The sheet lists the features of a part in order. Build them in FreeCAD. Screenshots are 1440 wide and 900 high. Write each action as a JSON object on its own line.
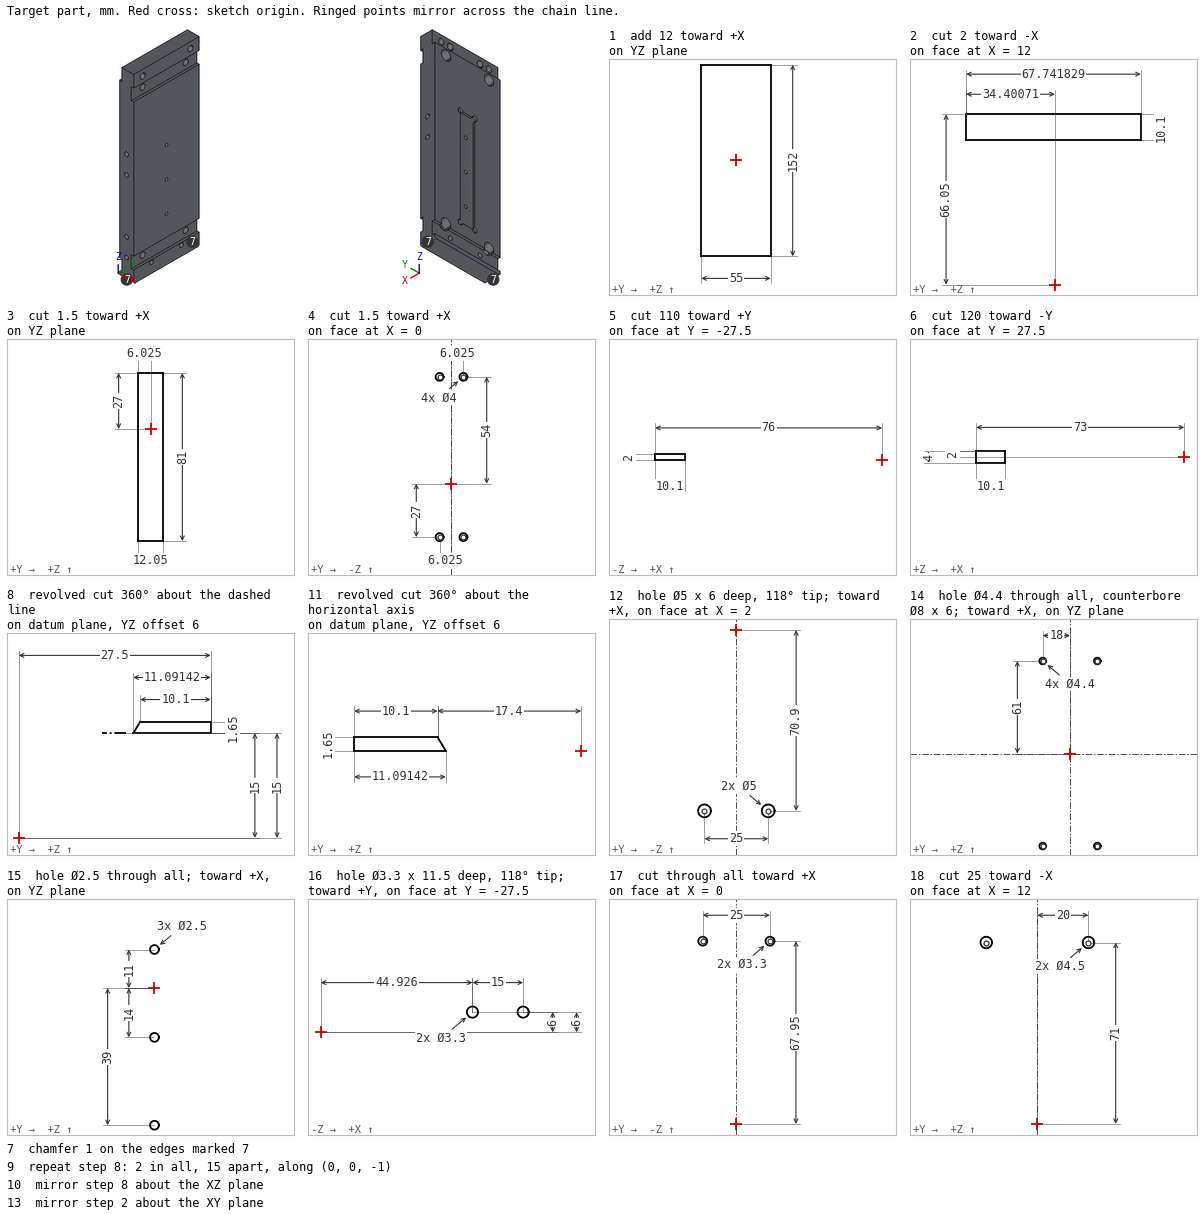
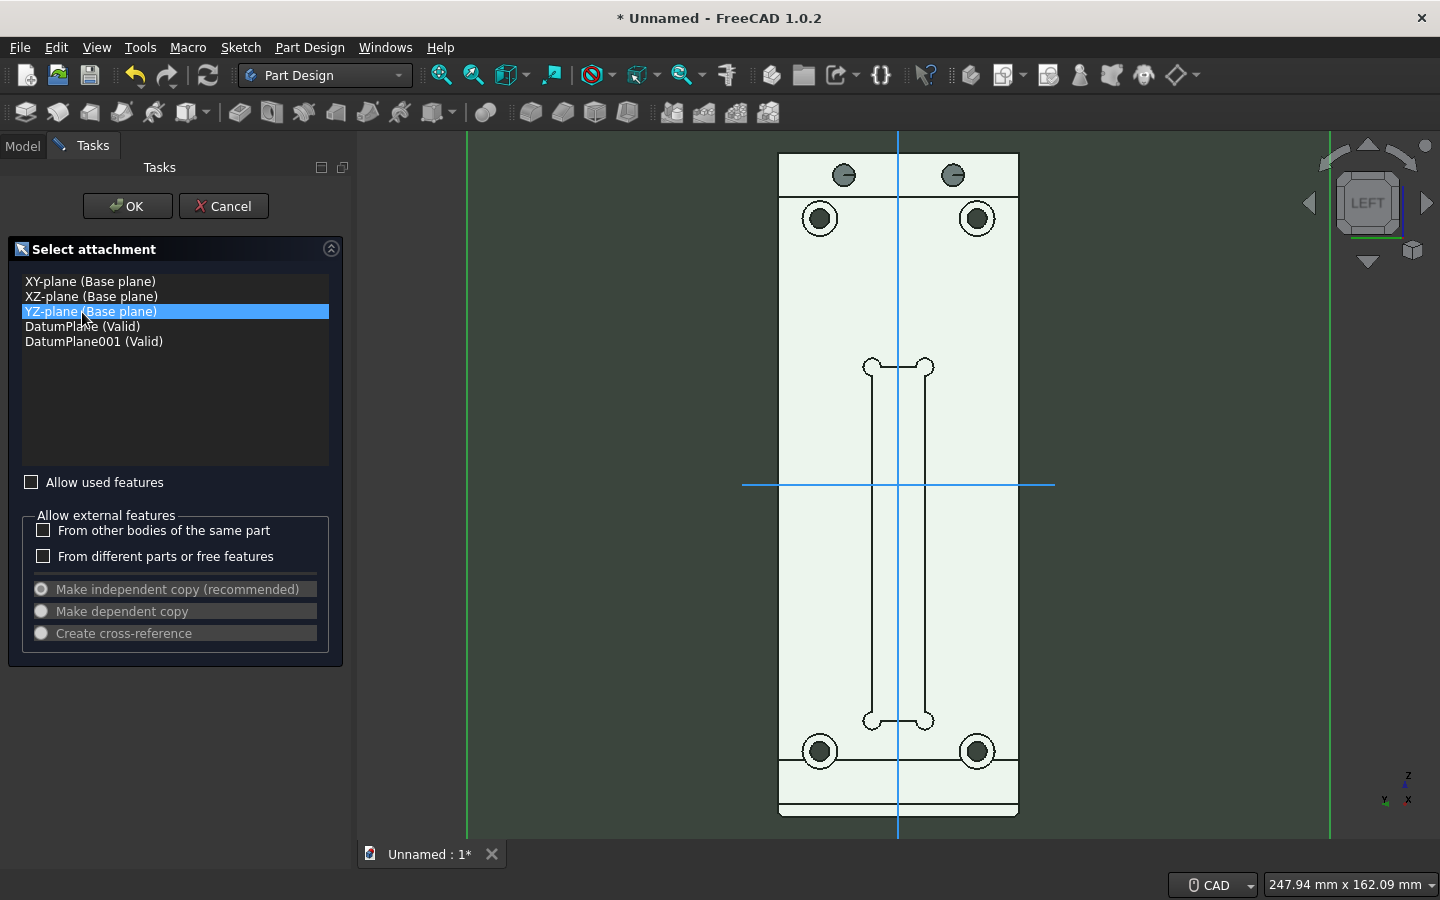
{"action": "left_click", "coordinate": [128, 206]}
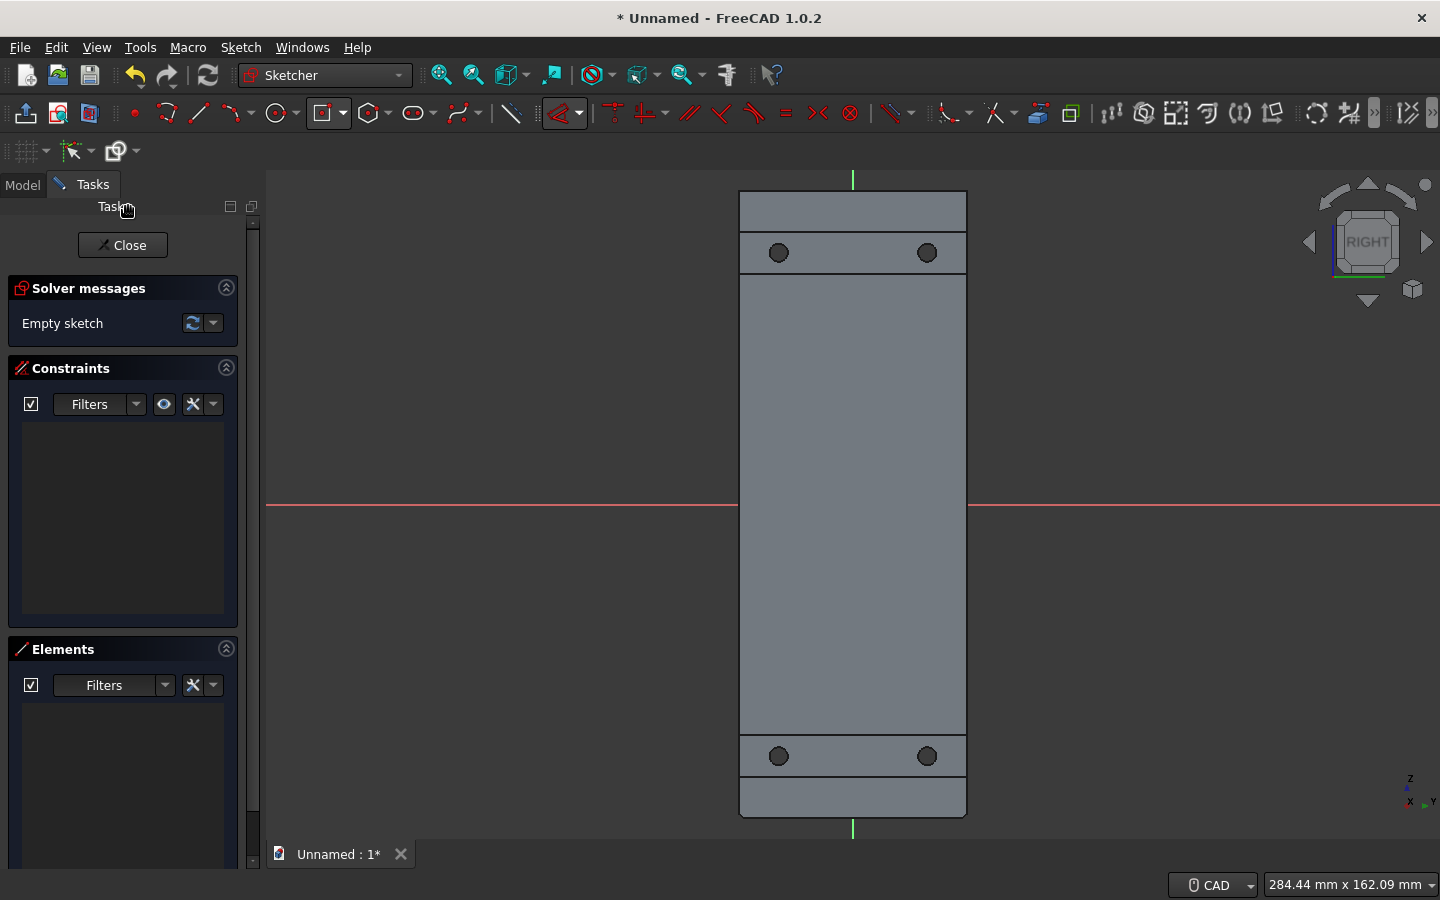
{"action": "key", "text": "q s"}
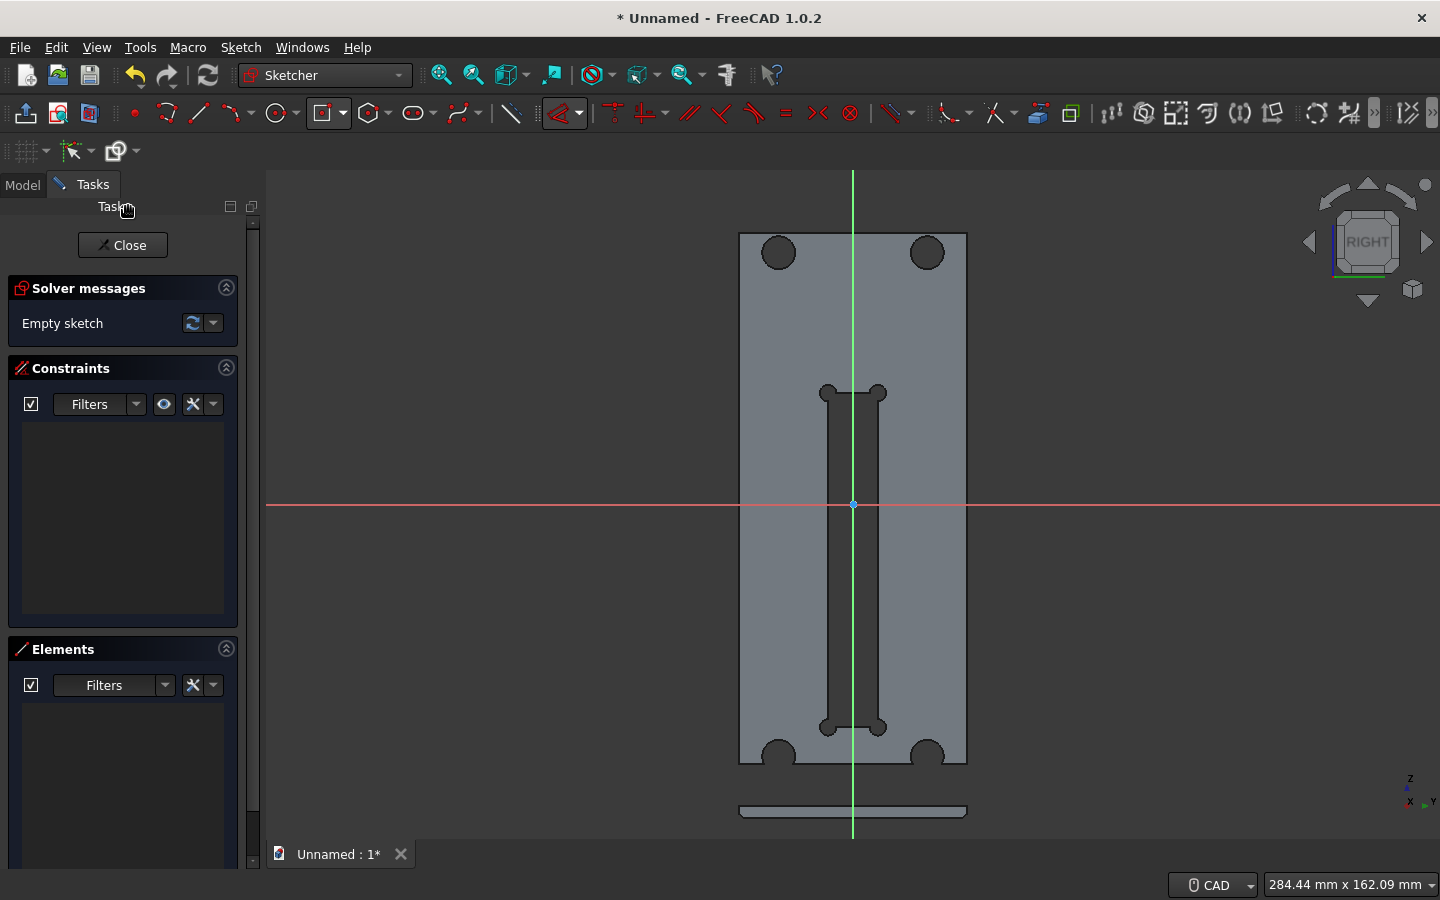
{"action": "scroll", "coordinate": [936, 633], "scroll_direction": "up", "scroll_amount": 3}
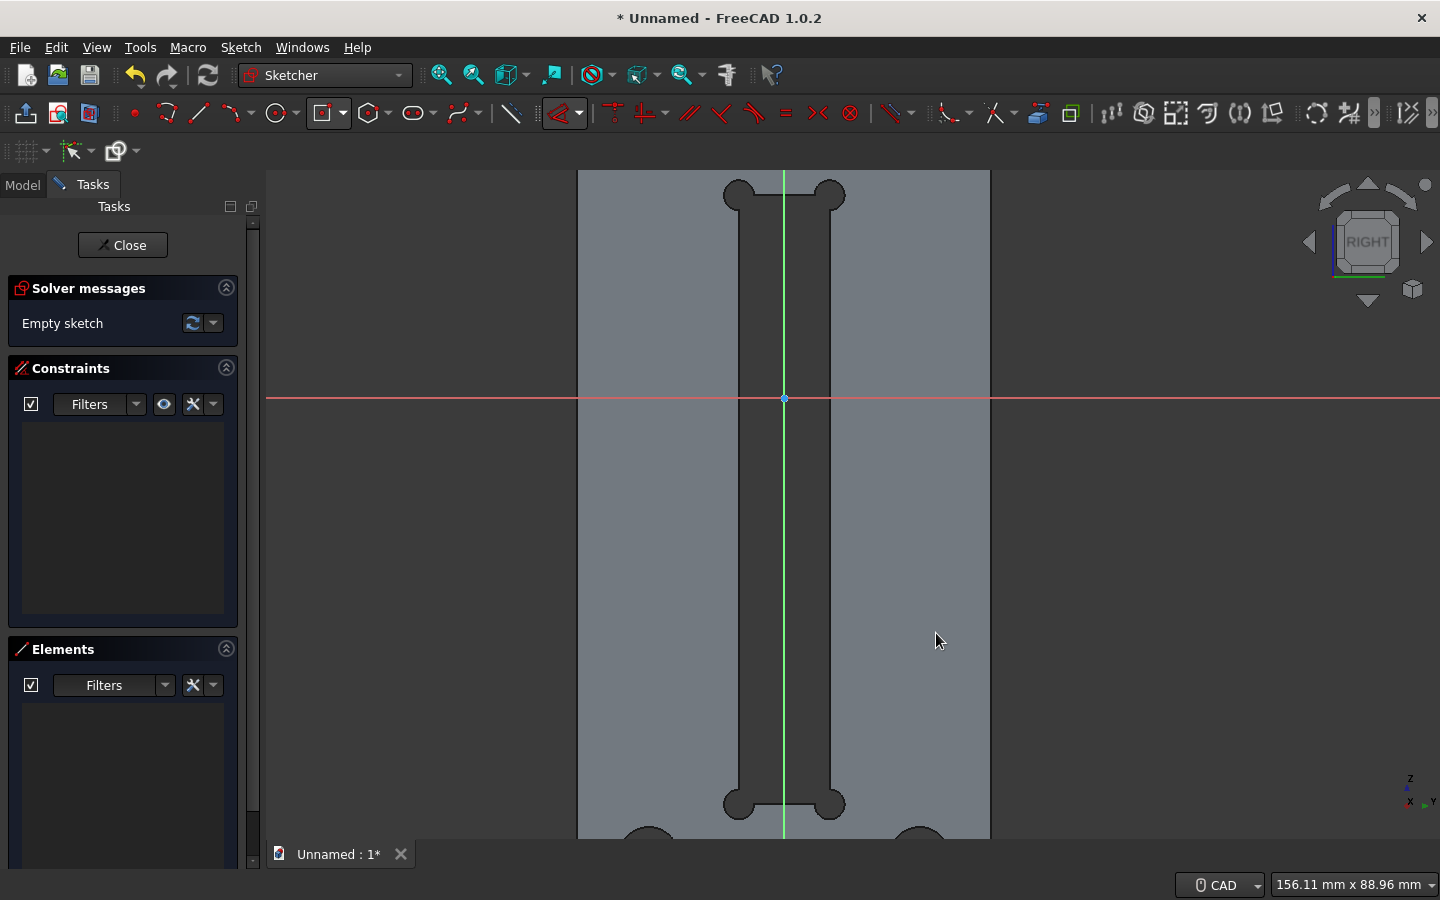
{"action": "left_click", "coordinate": [276, 114]}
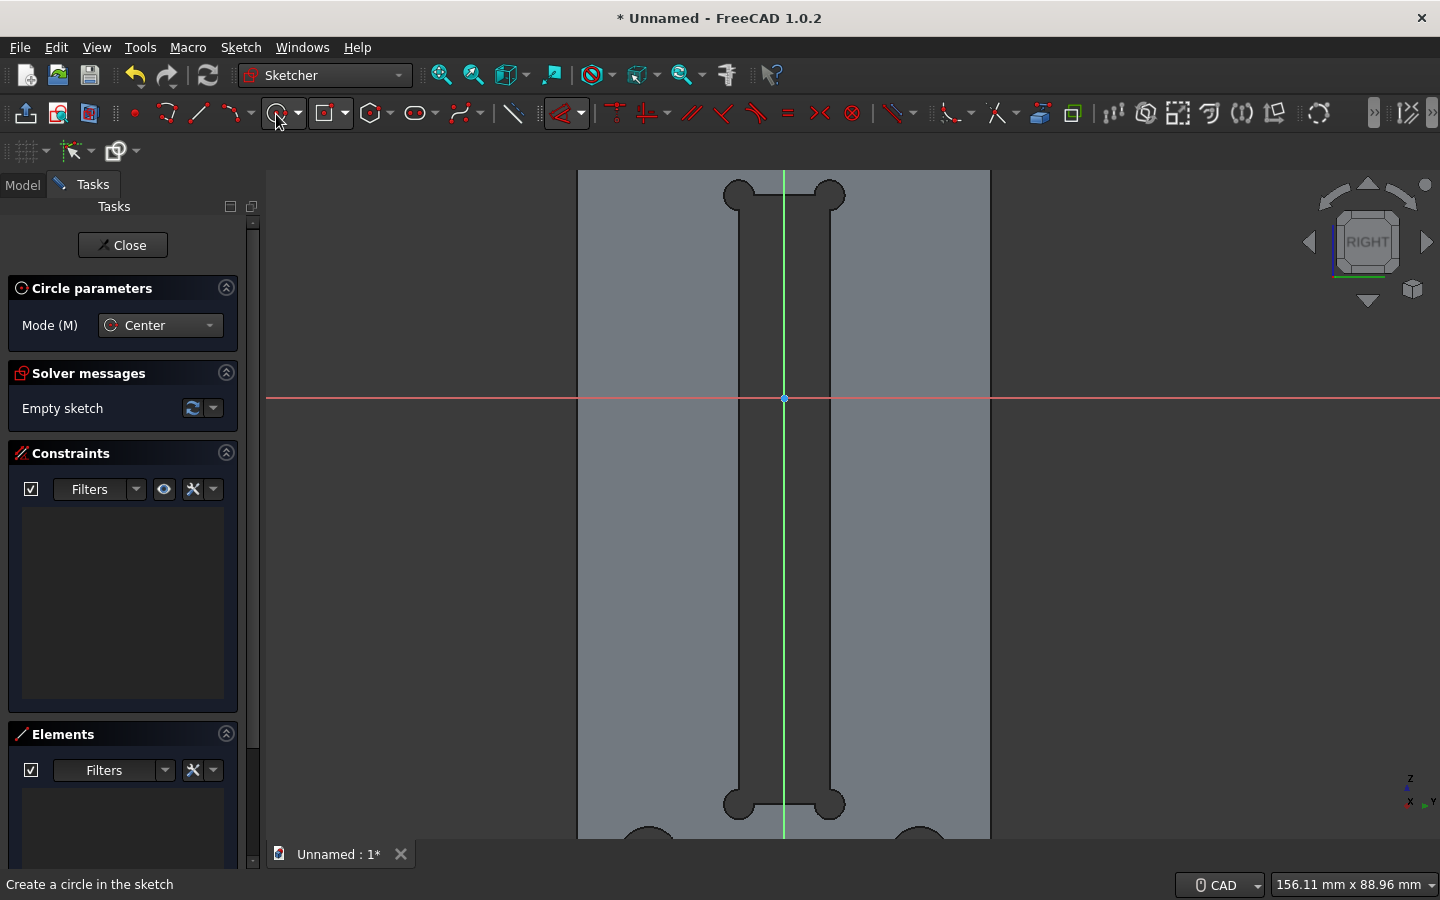
{"action": "scroll", "coordinate": [784, 316], "scroll_direction": "up", "scroll_amount": 5}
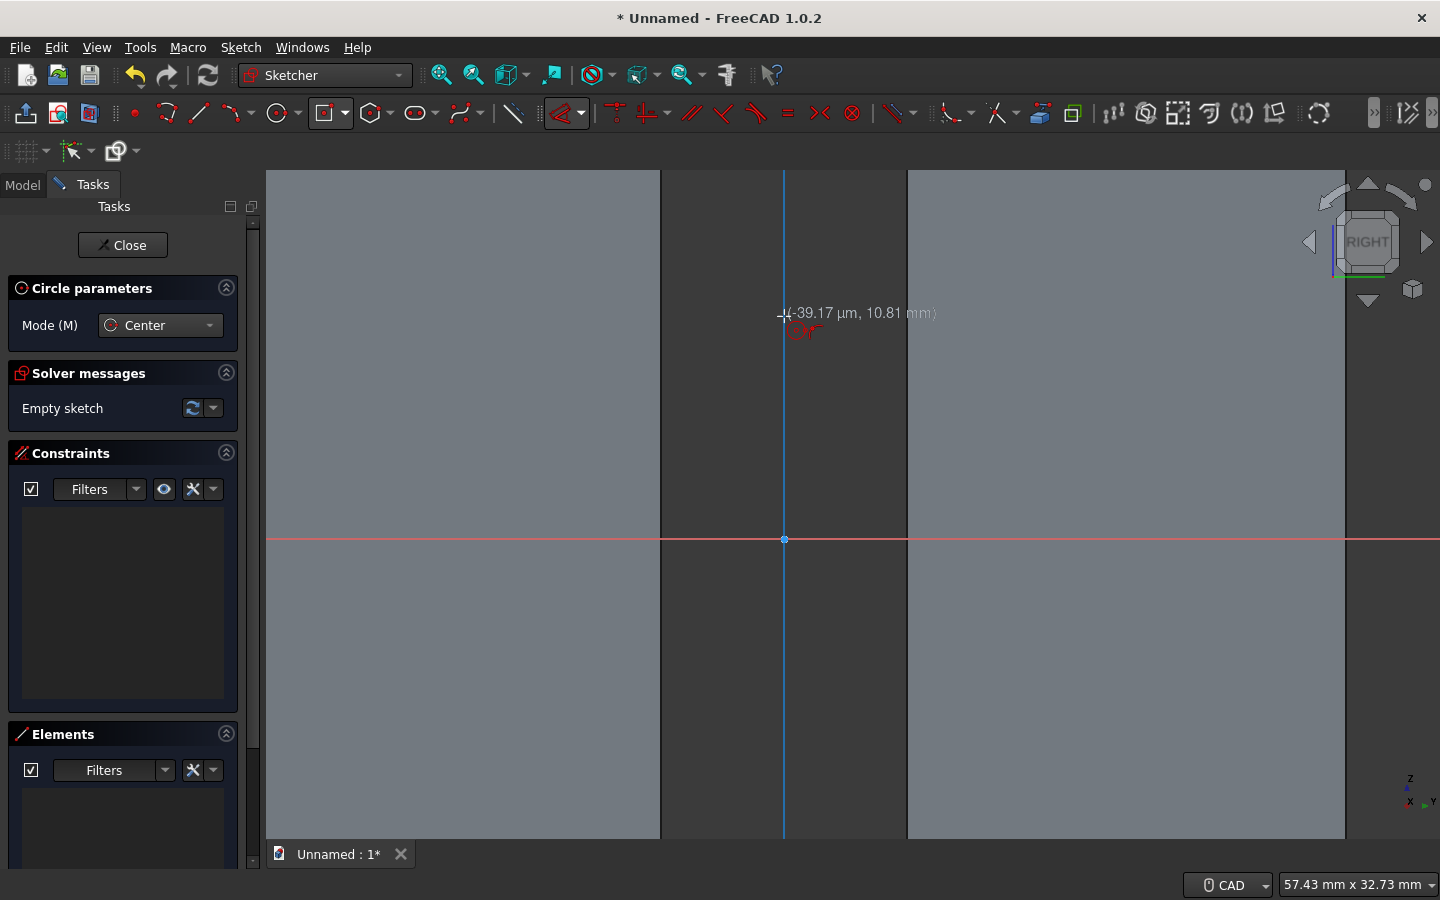
{"action": "left_click", "coordinate": [784, 314]}
{"action": "mouse_move", "coordinate": [802, 296]}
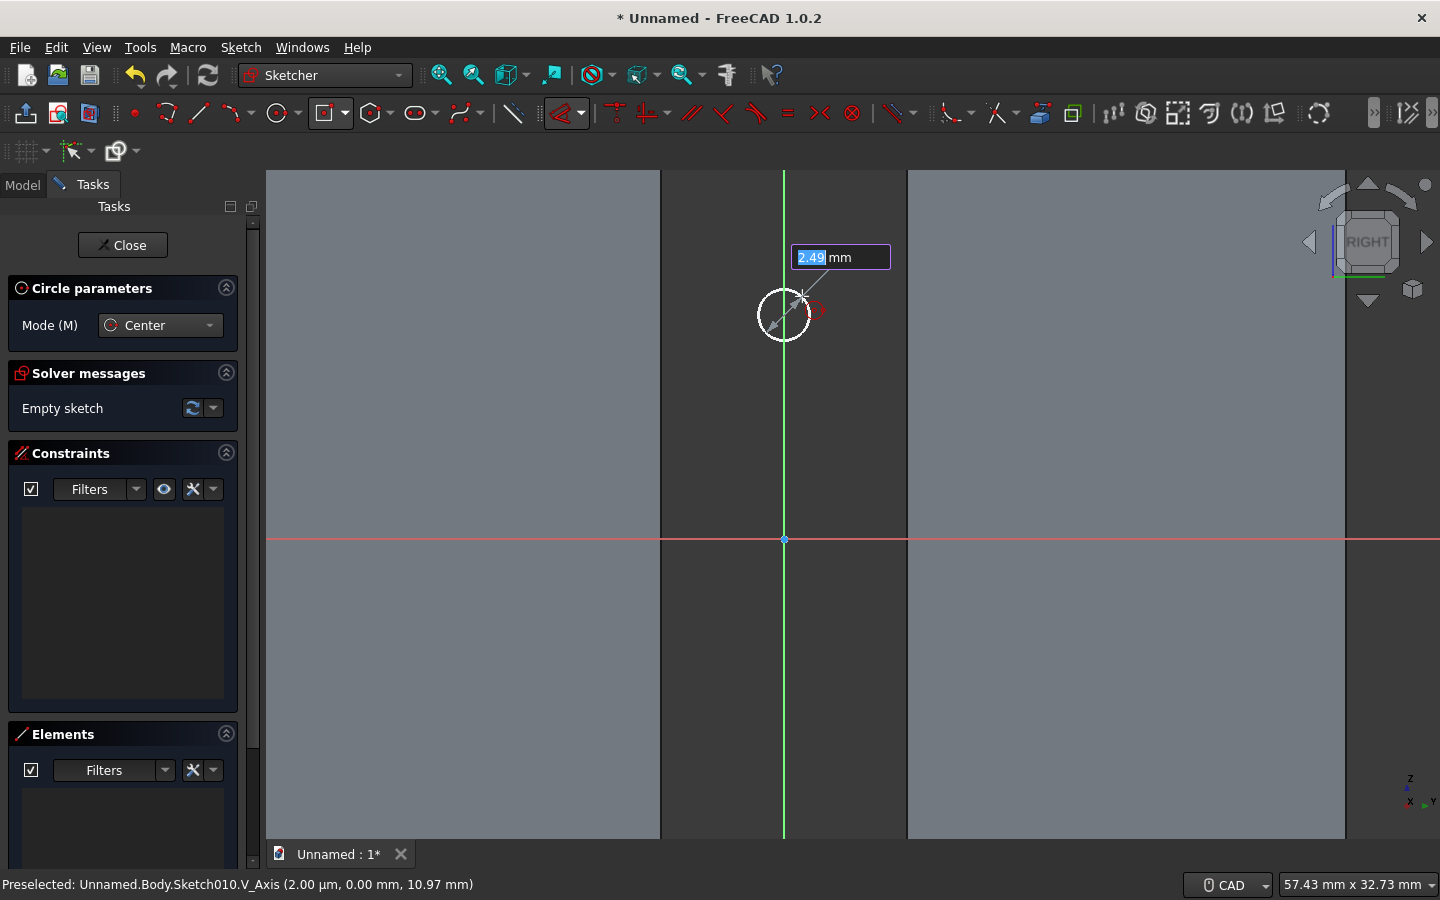
{"action": "type", "text": "2.5"}
{"action": "key", "text": "Return"}